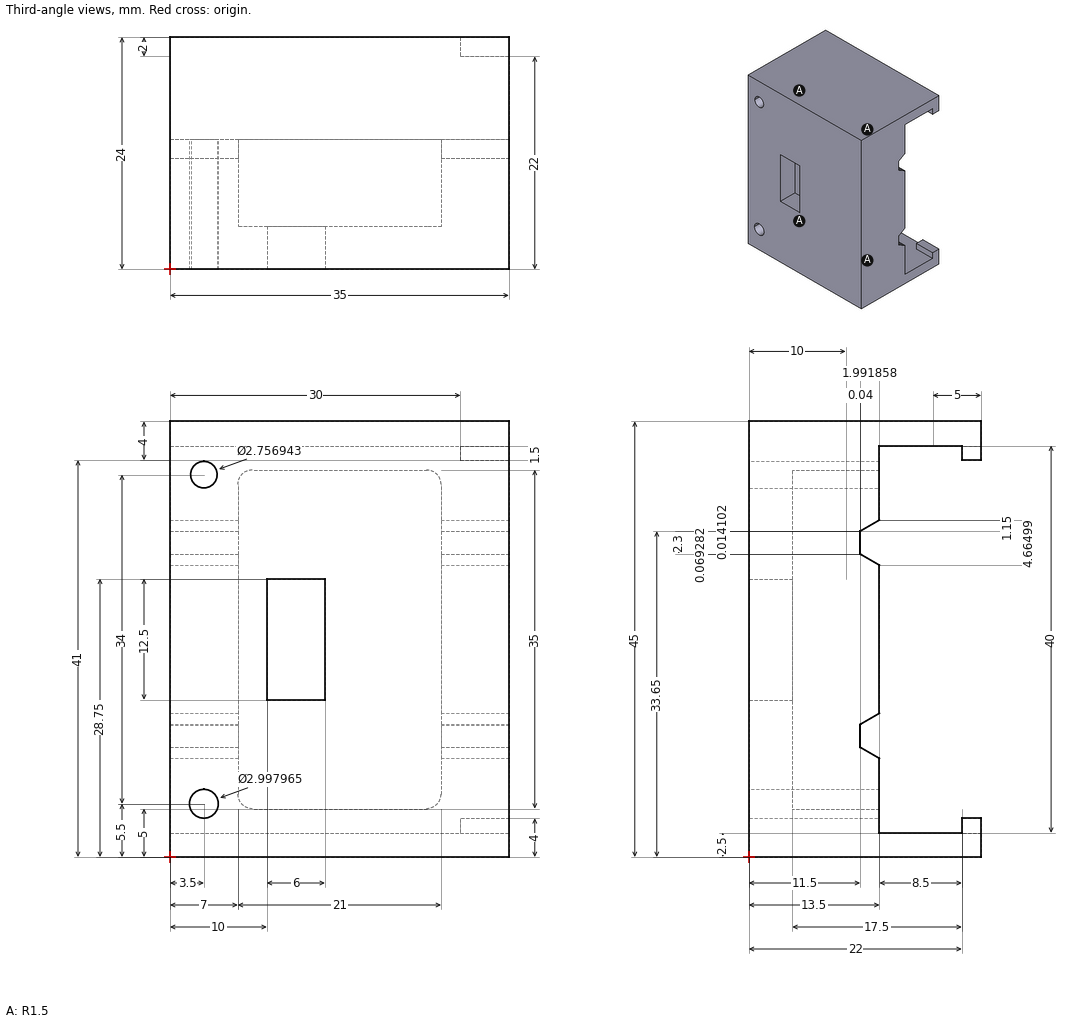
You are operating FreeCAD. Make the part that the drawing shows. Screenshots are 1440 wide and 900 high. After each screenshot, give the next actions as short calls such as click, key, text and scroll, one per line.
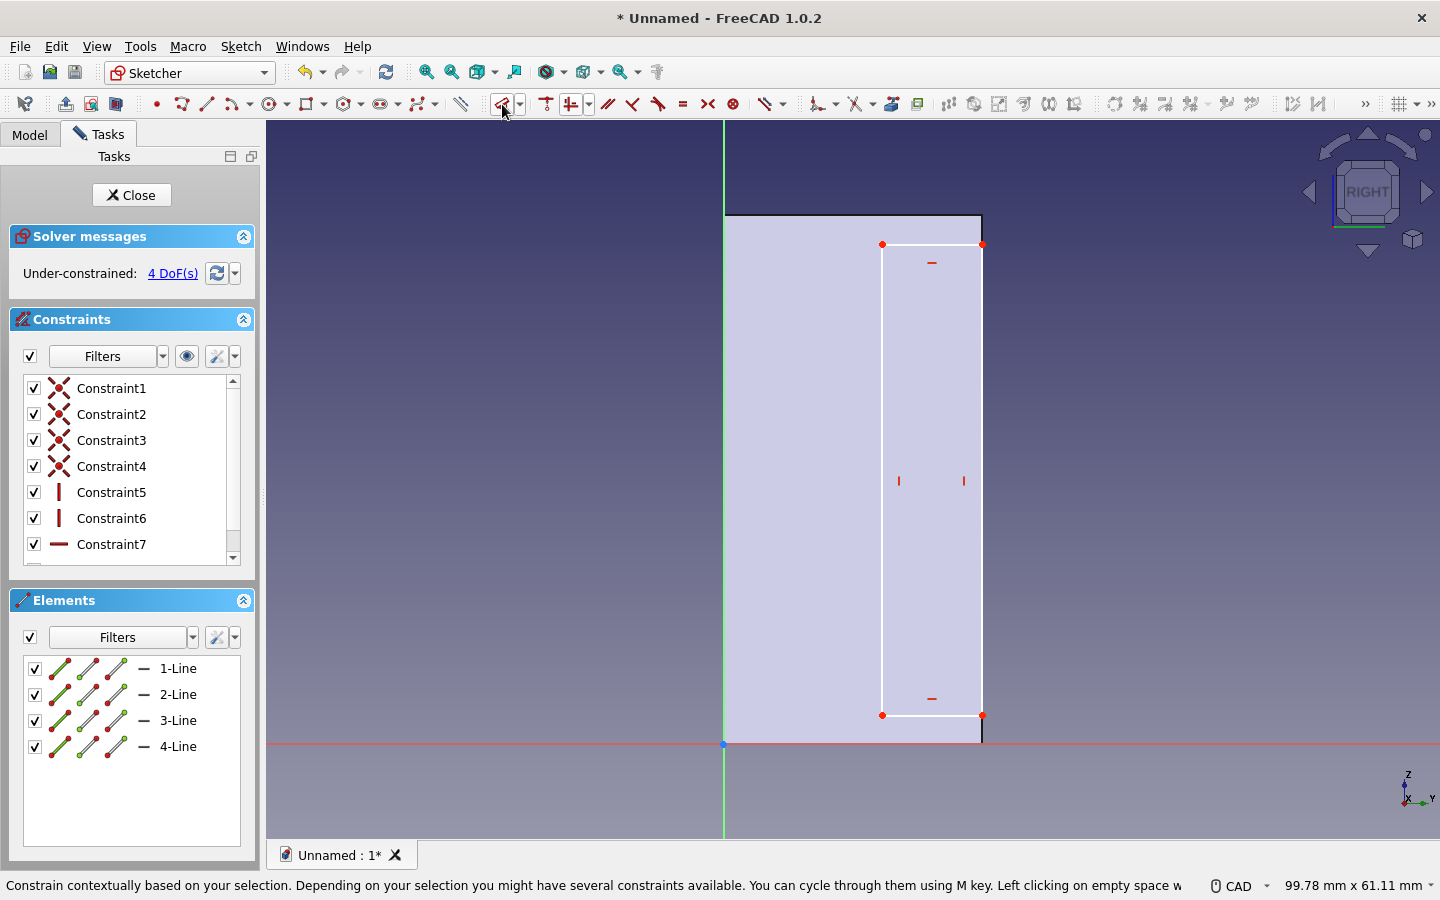
click(882, 386)
click(916, 481)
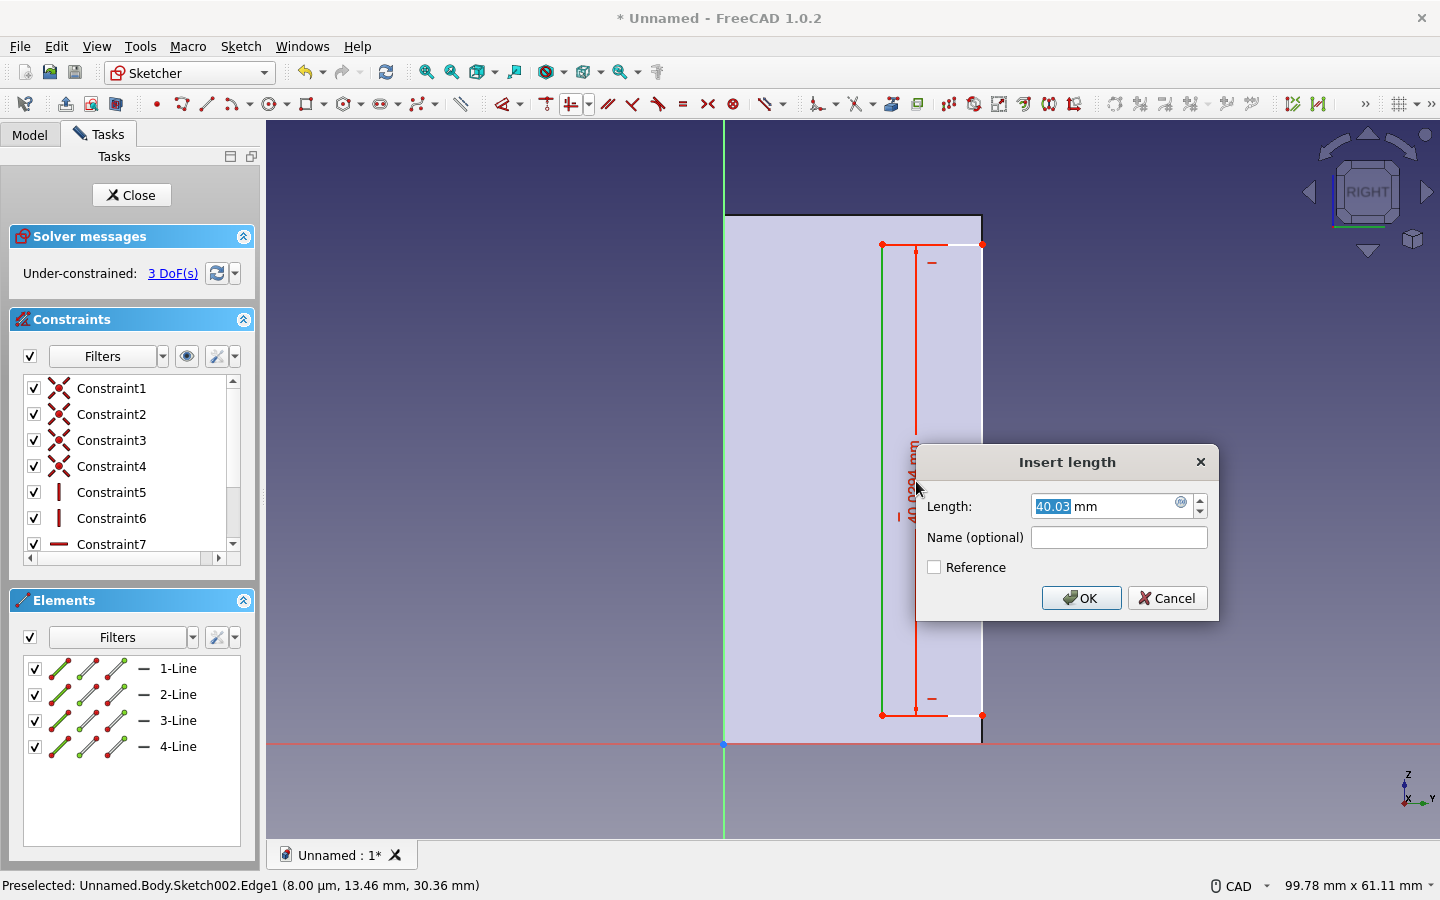
text(40)
key(Return)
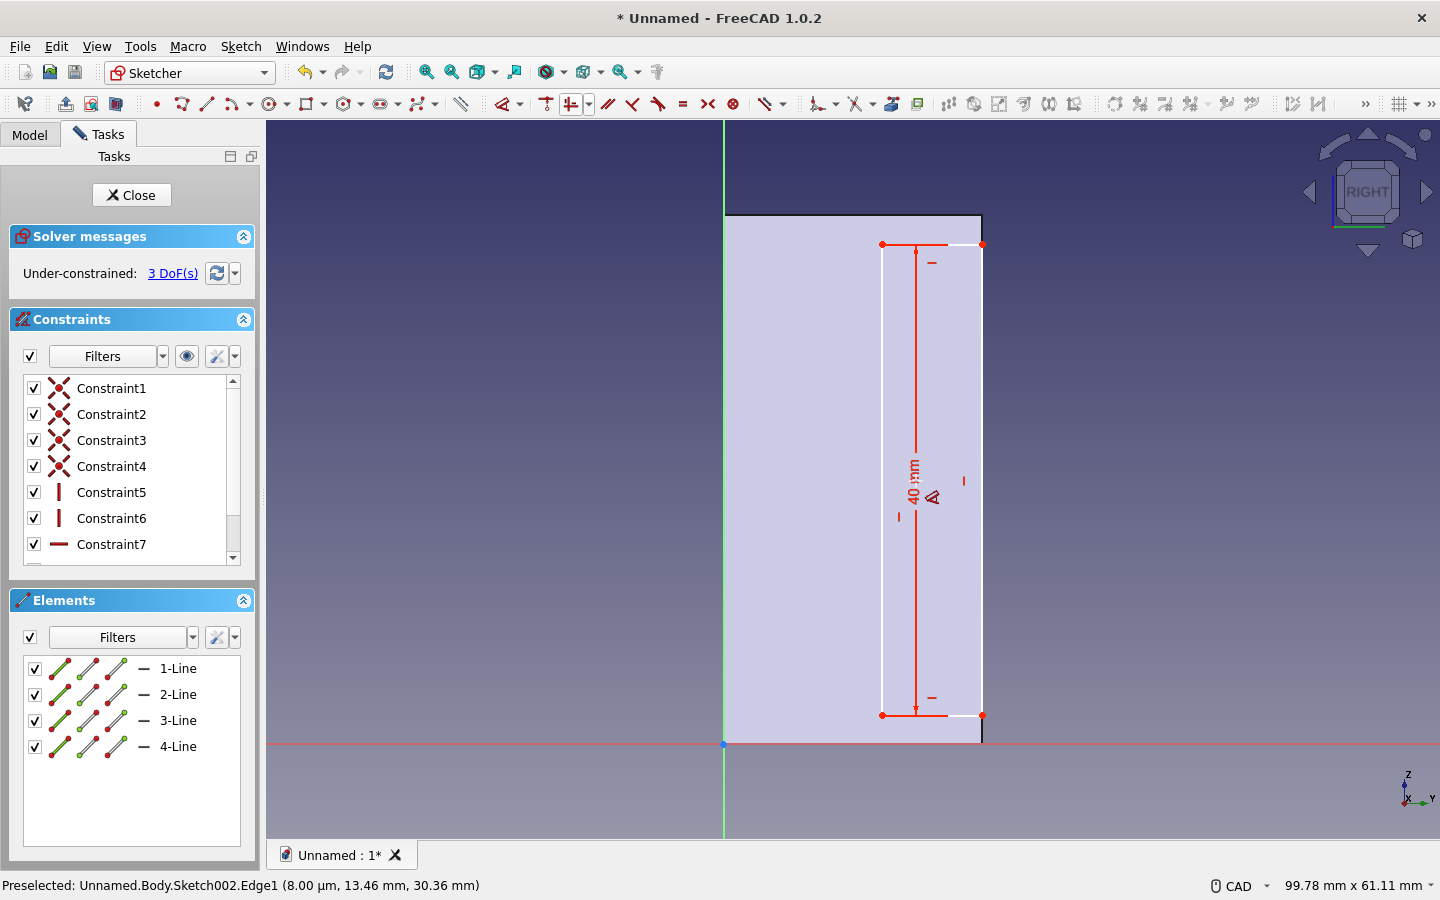
click(912, 716)
click(932, 682)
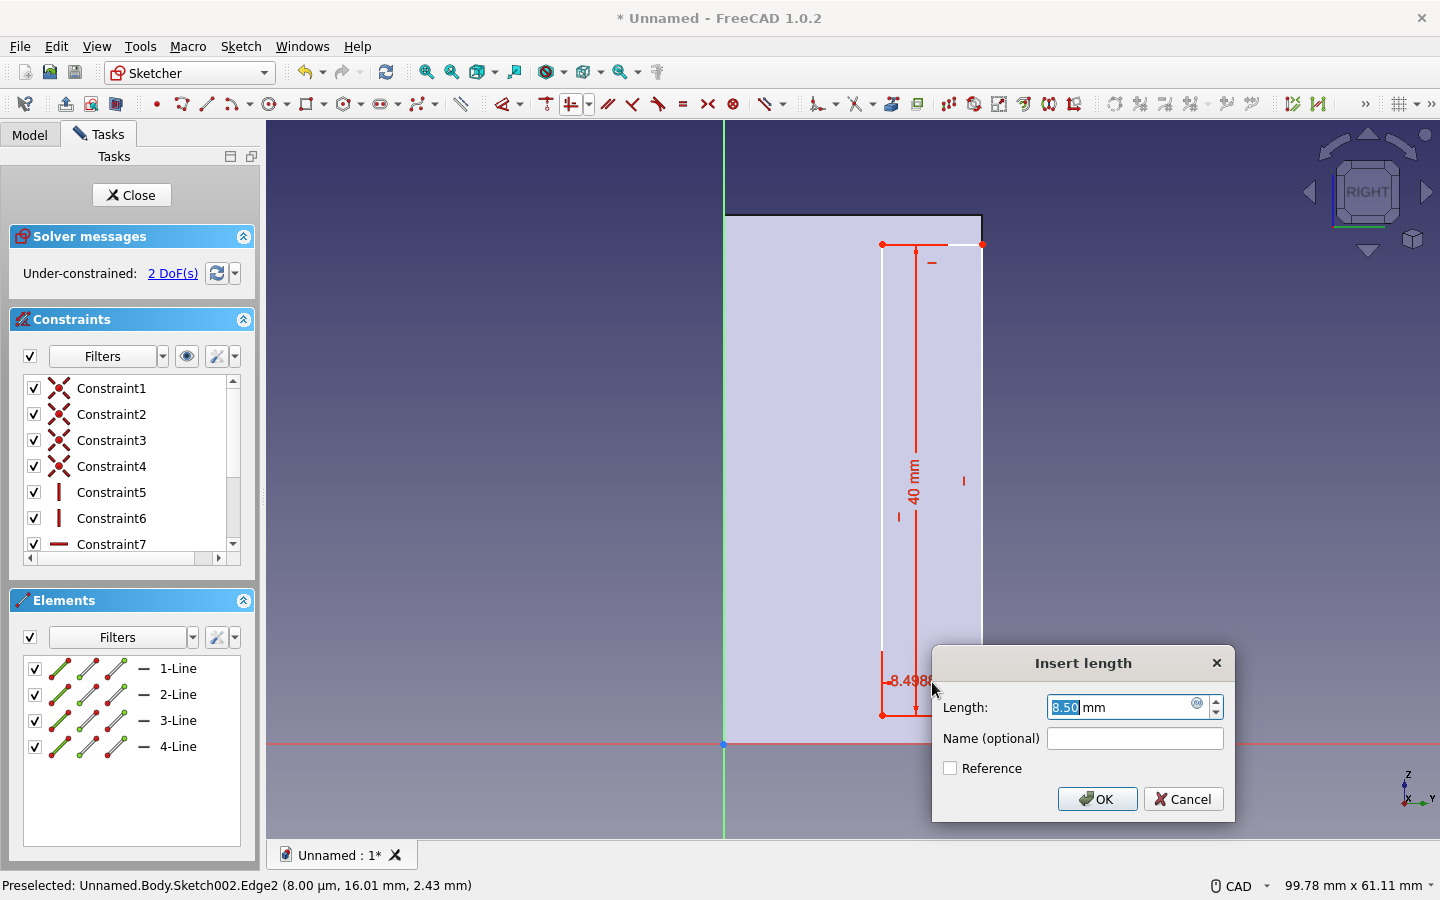
text(8.5)
key(Return)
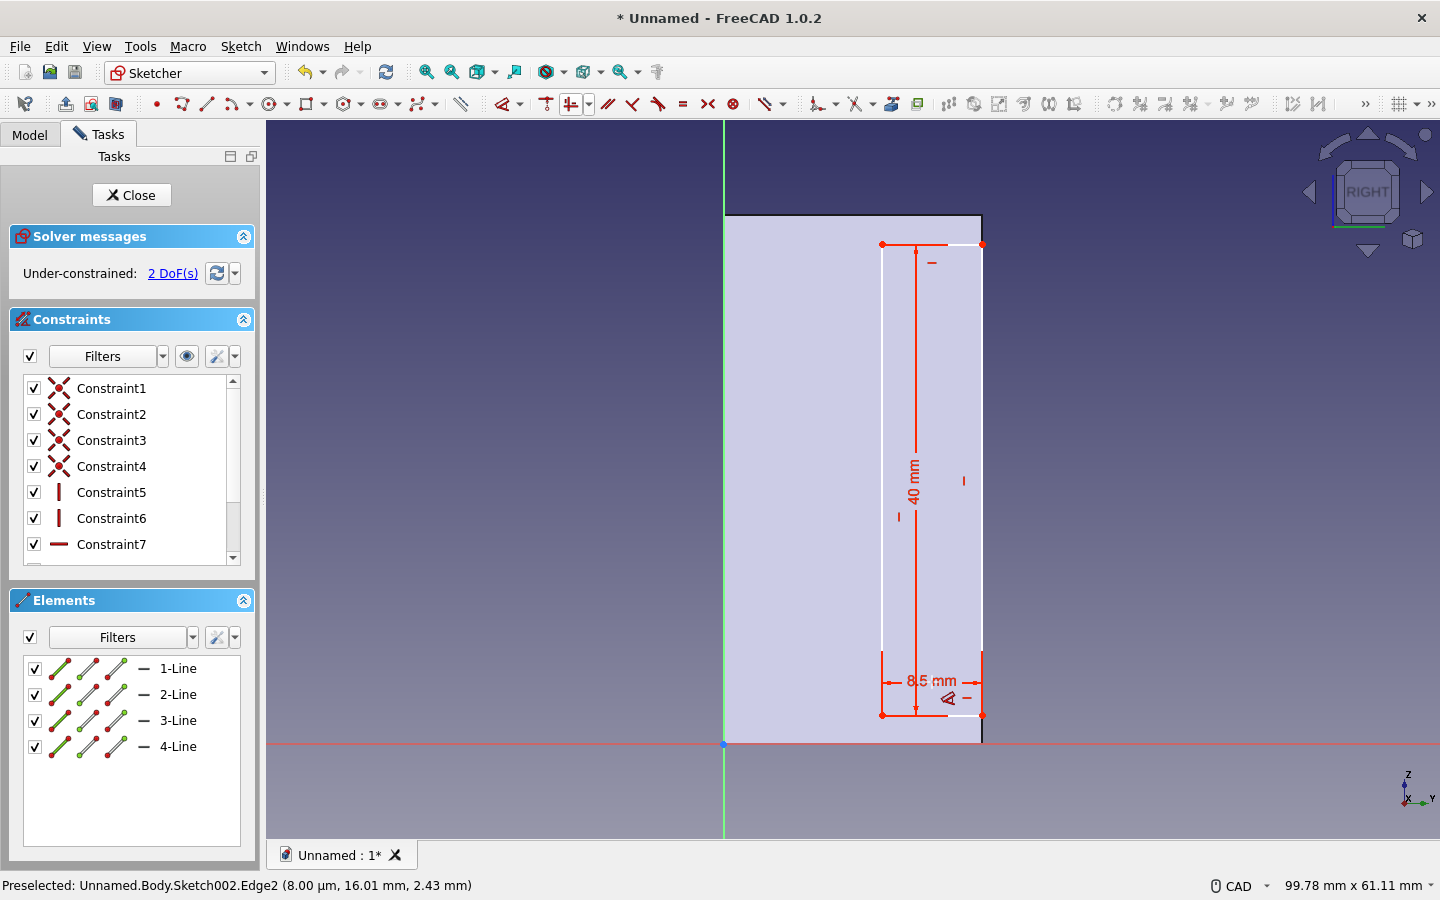
click(982, 716)
click(853, 778)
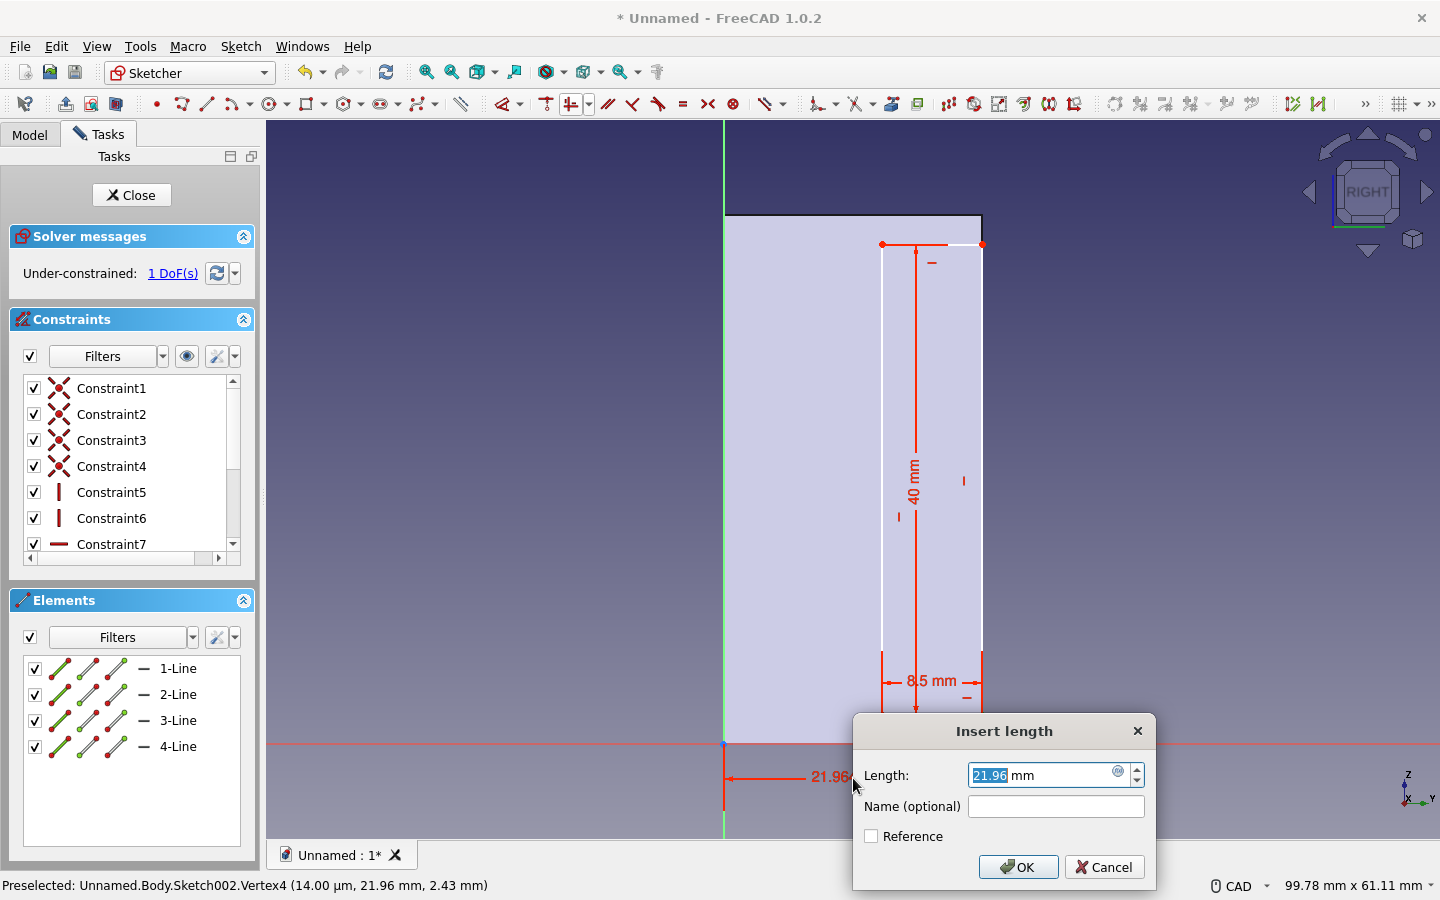
text(22)
key(Return)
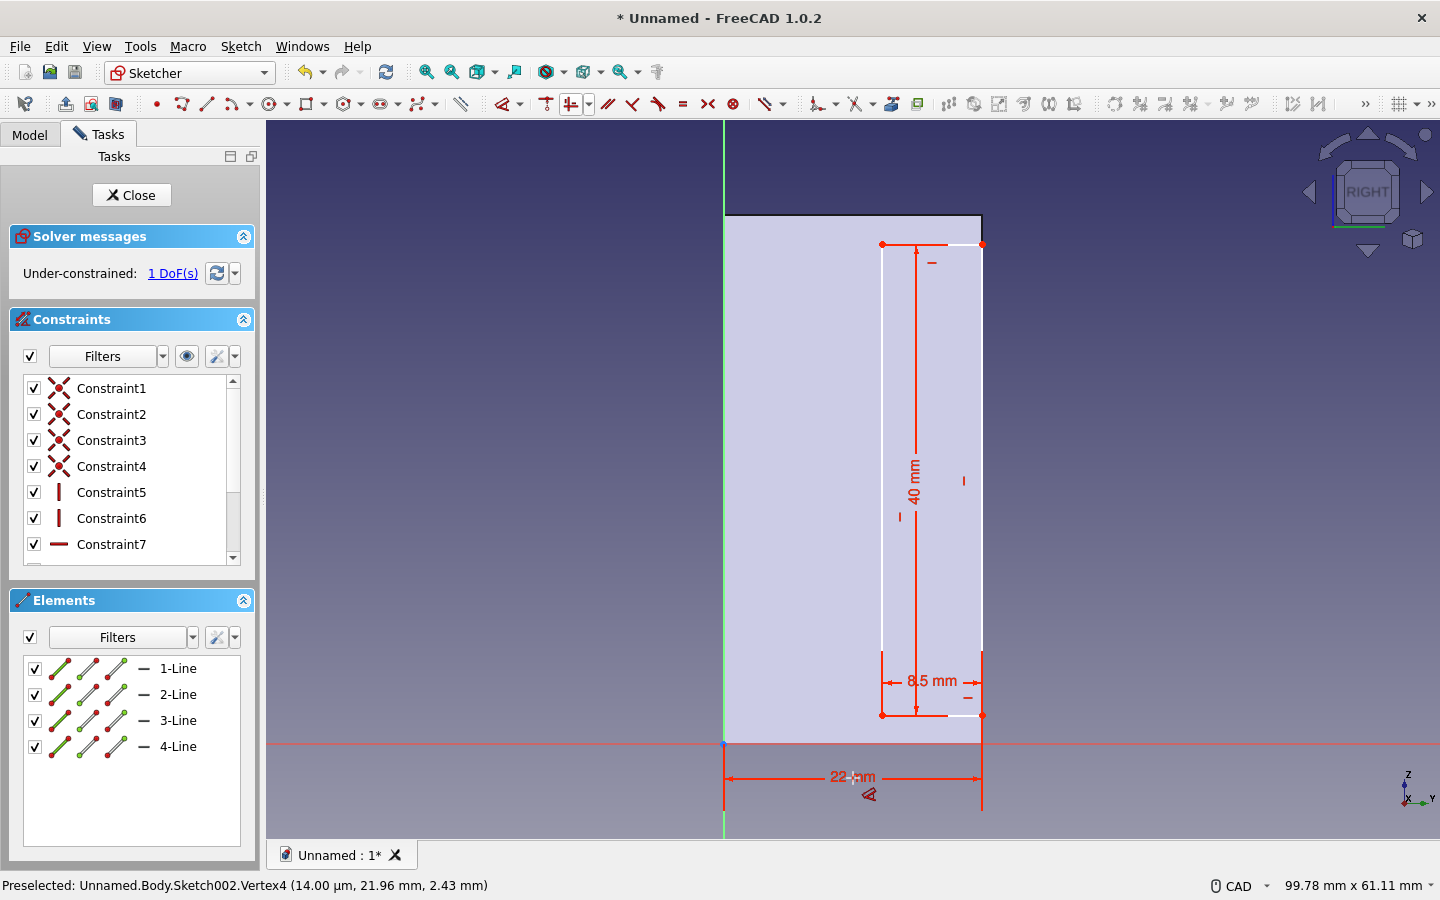
scroll(882, 716, up, 2)